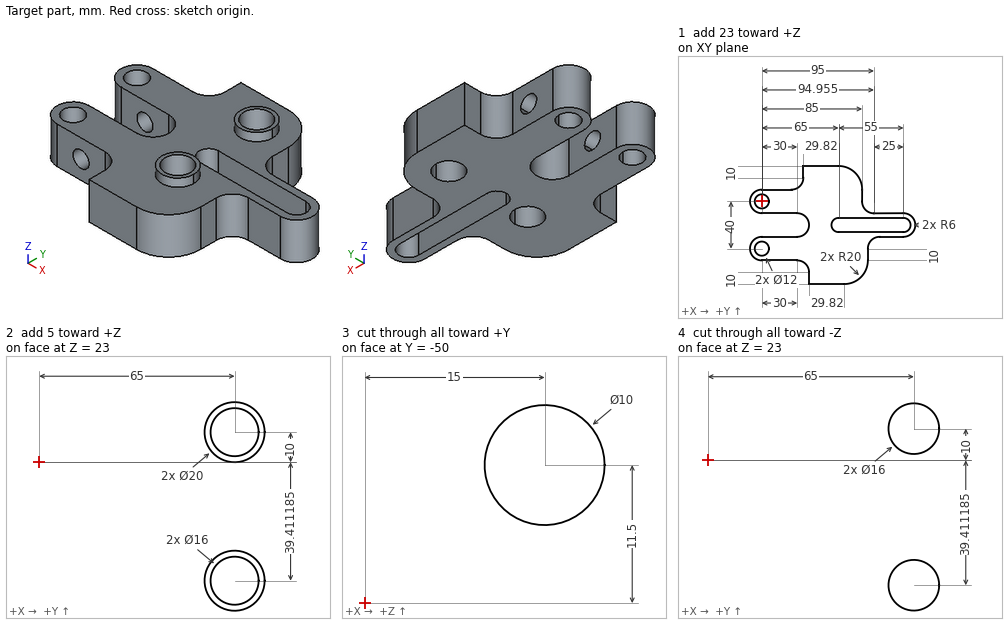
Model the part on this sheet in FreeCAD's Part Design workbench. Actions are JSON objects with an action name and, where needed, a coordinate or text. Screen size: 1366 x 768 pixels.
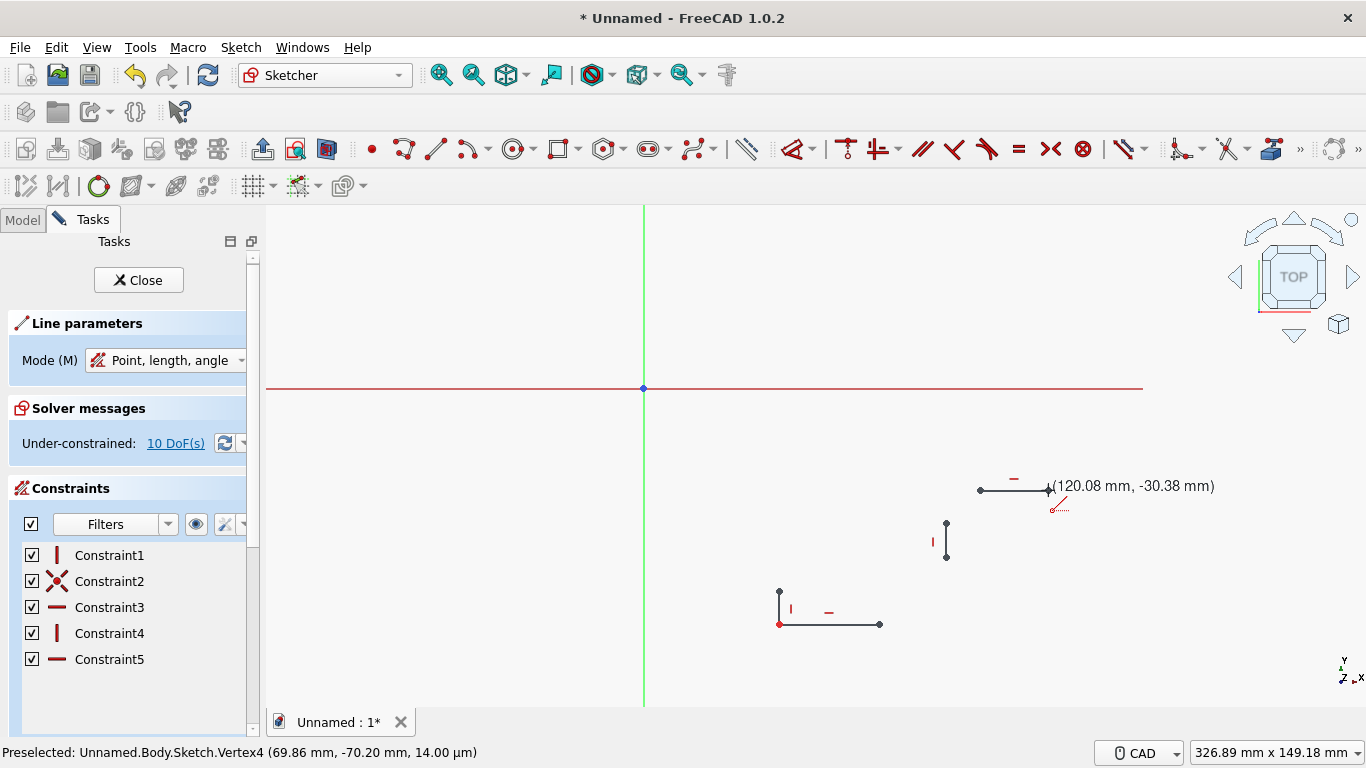
{"action": "left_click", "coordinate": [1048, 422]}
{"action": "left_click", "coordinate": [964, 427]}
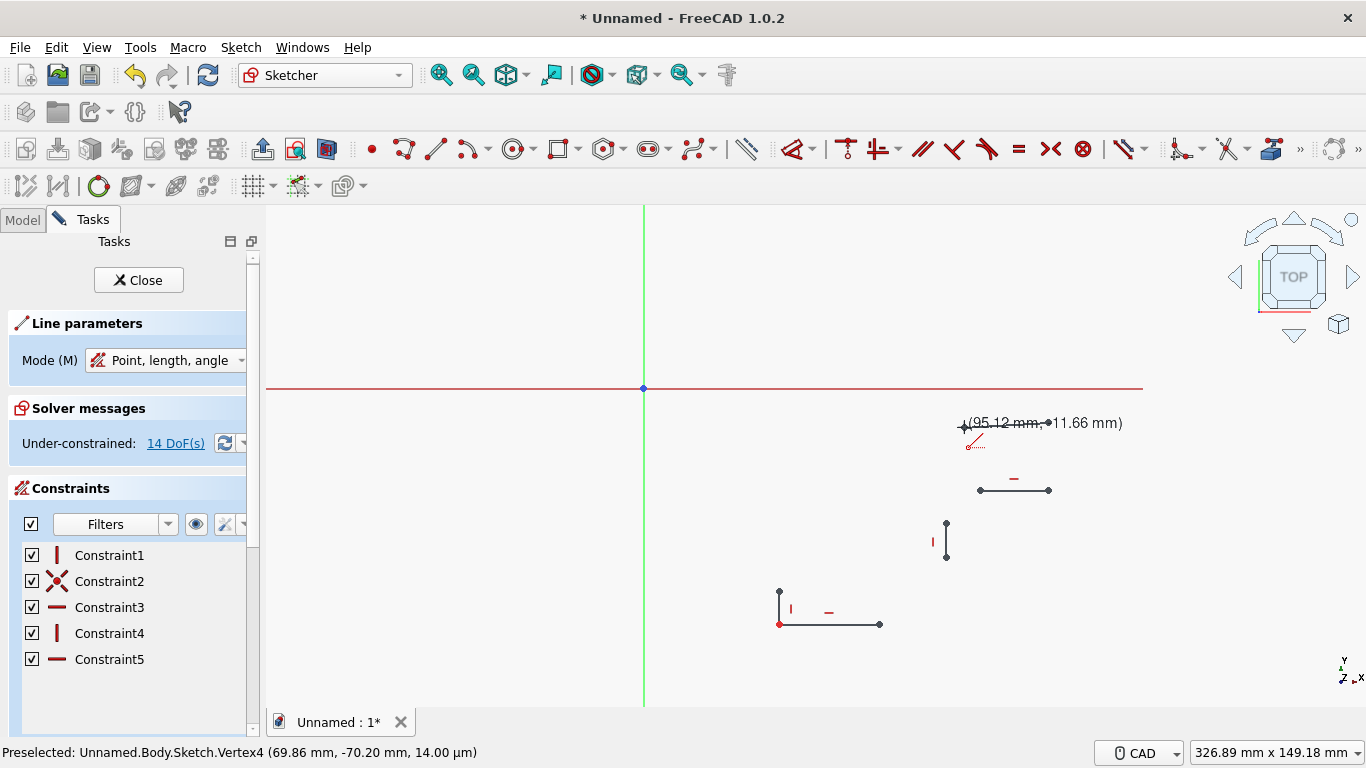
{"action": "scroll", "coordinate": [930, 389], "scroll_direction": "up", "scroll_amount": 22}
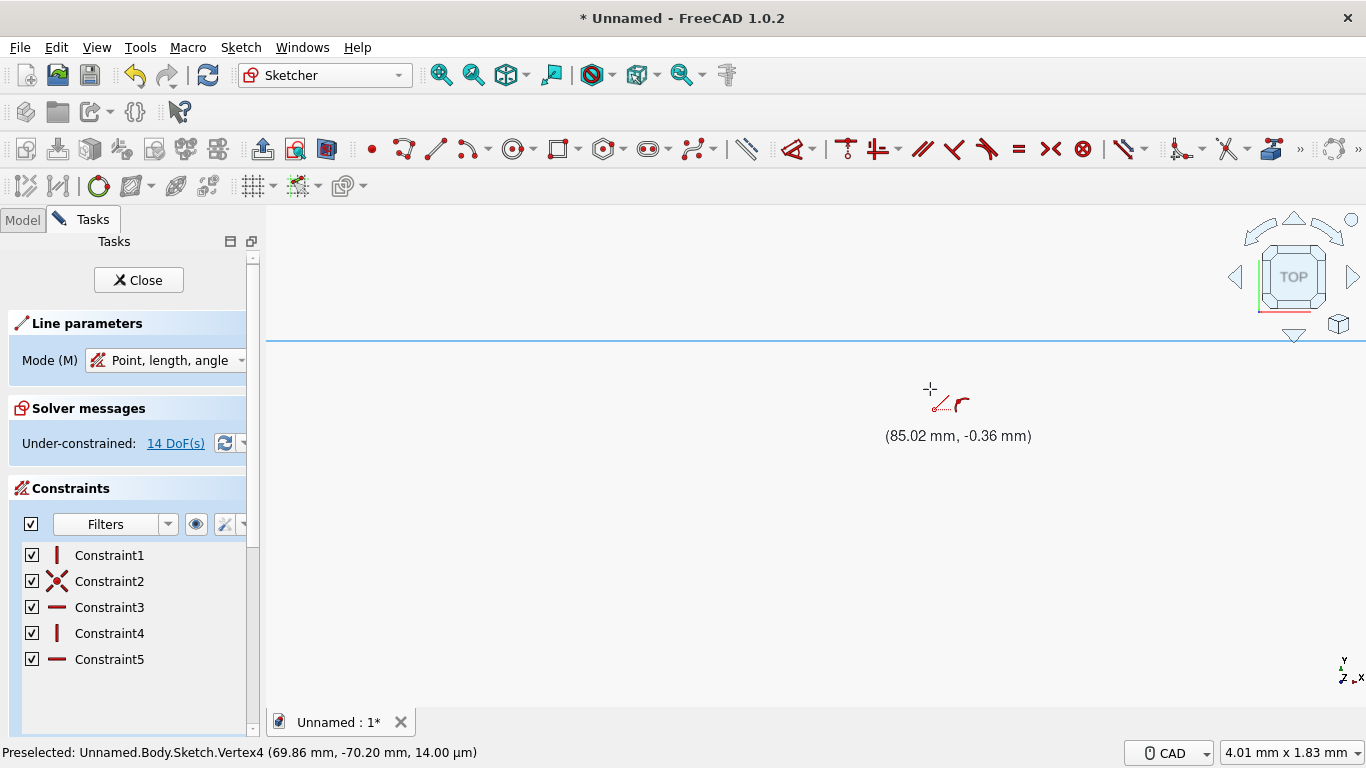
{"action": "left_click", "coordinate": [864, 360]}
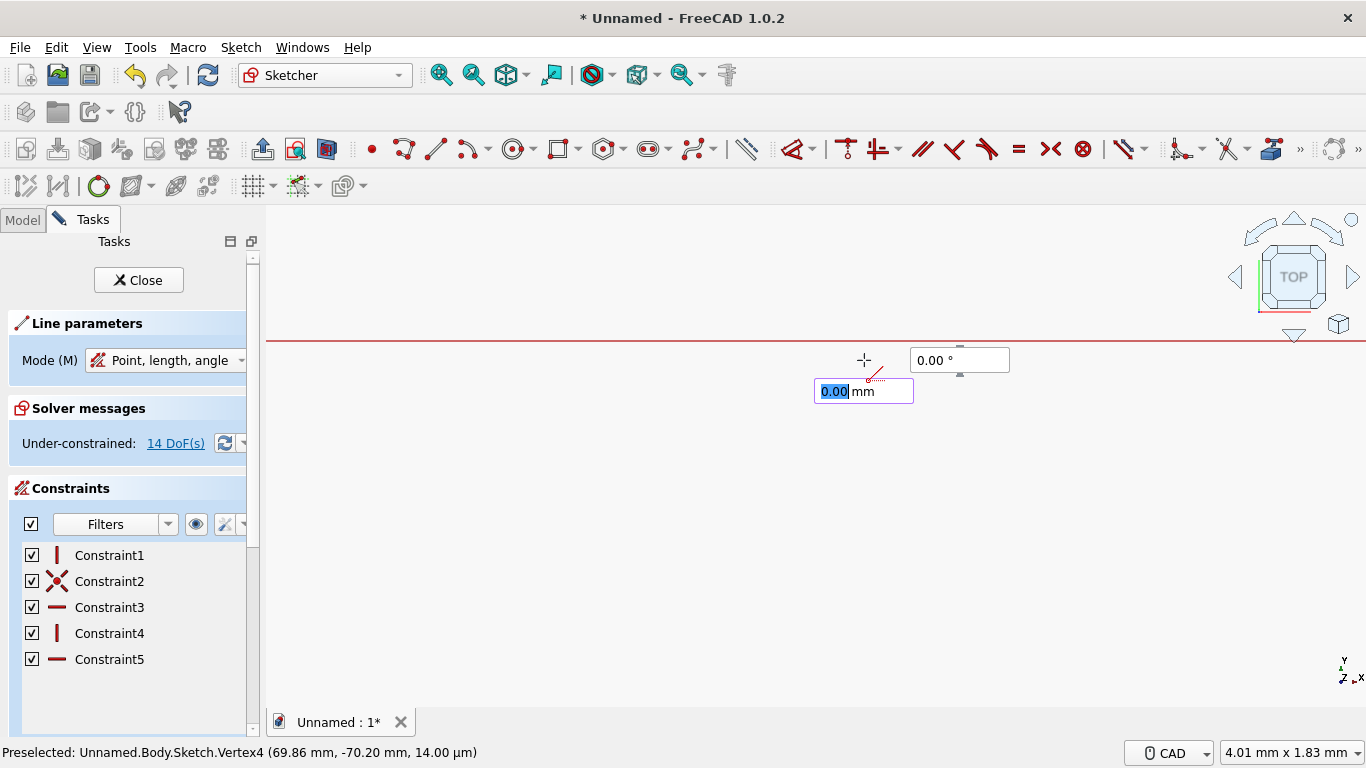
{"action": "scroll", "coordinate": [748, 456], "scroll_direction": "down", "scroll_amount": 15}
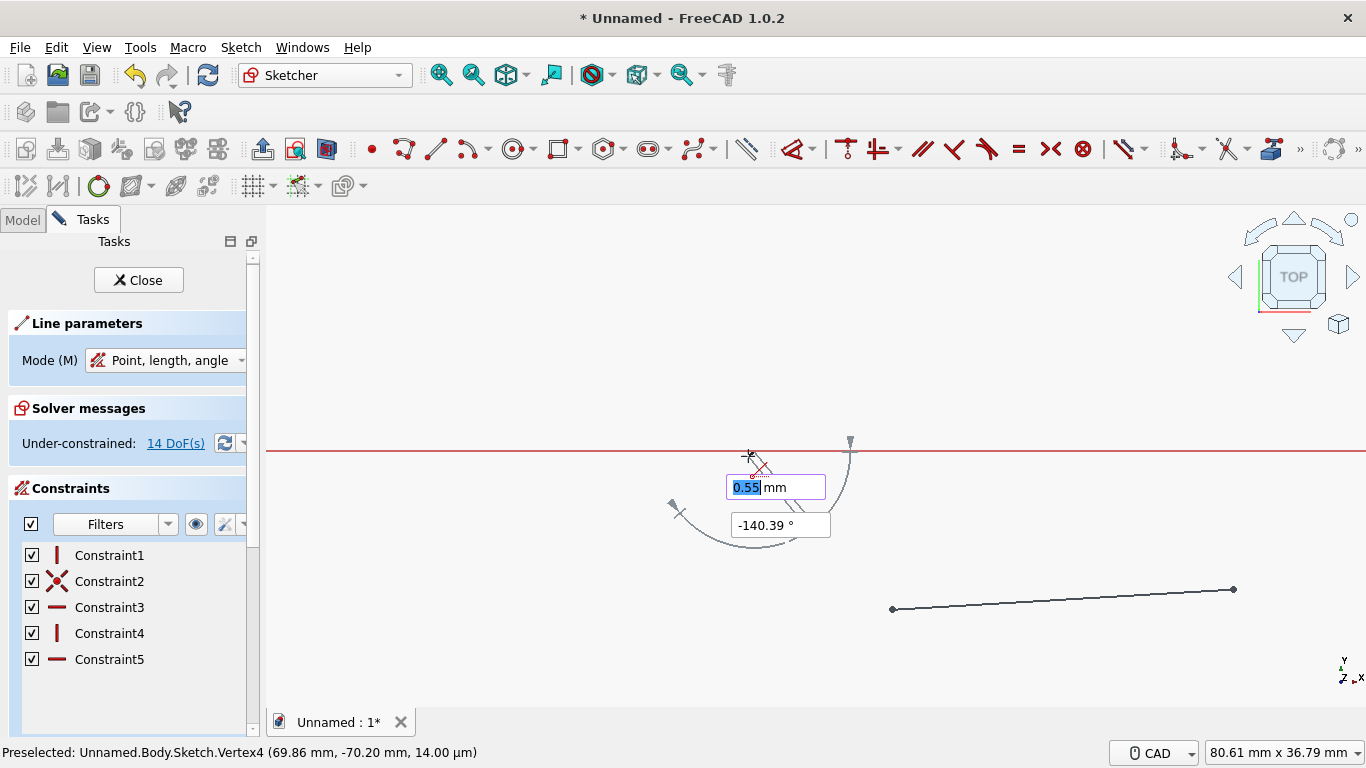
{"action": "scroll", "coordinate": [857, 368], "scroll_direction": "down", "scroll_amount": 7}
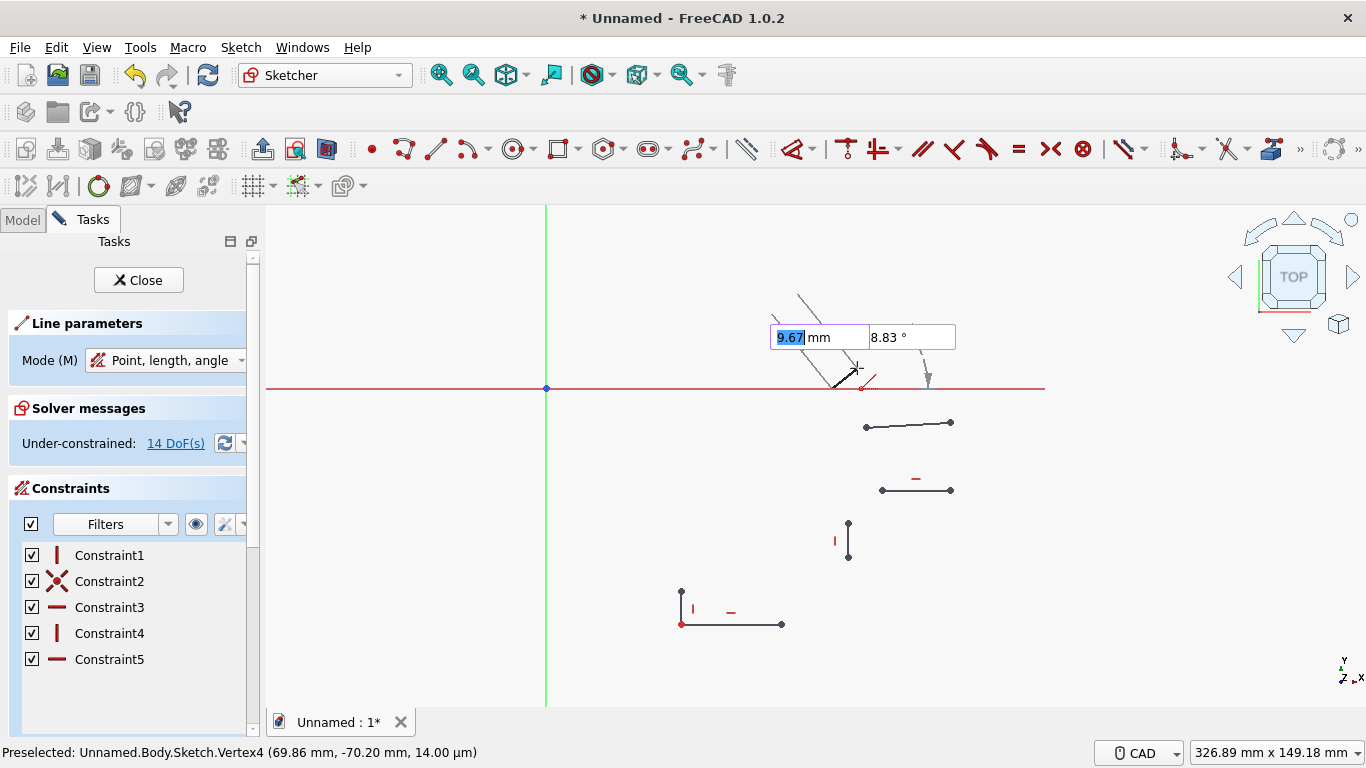
{"action": "left_click", "coordinate": [835, 355]}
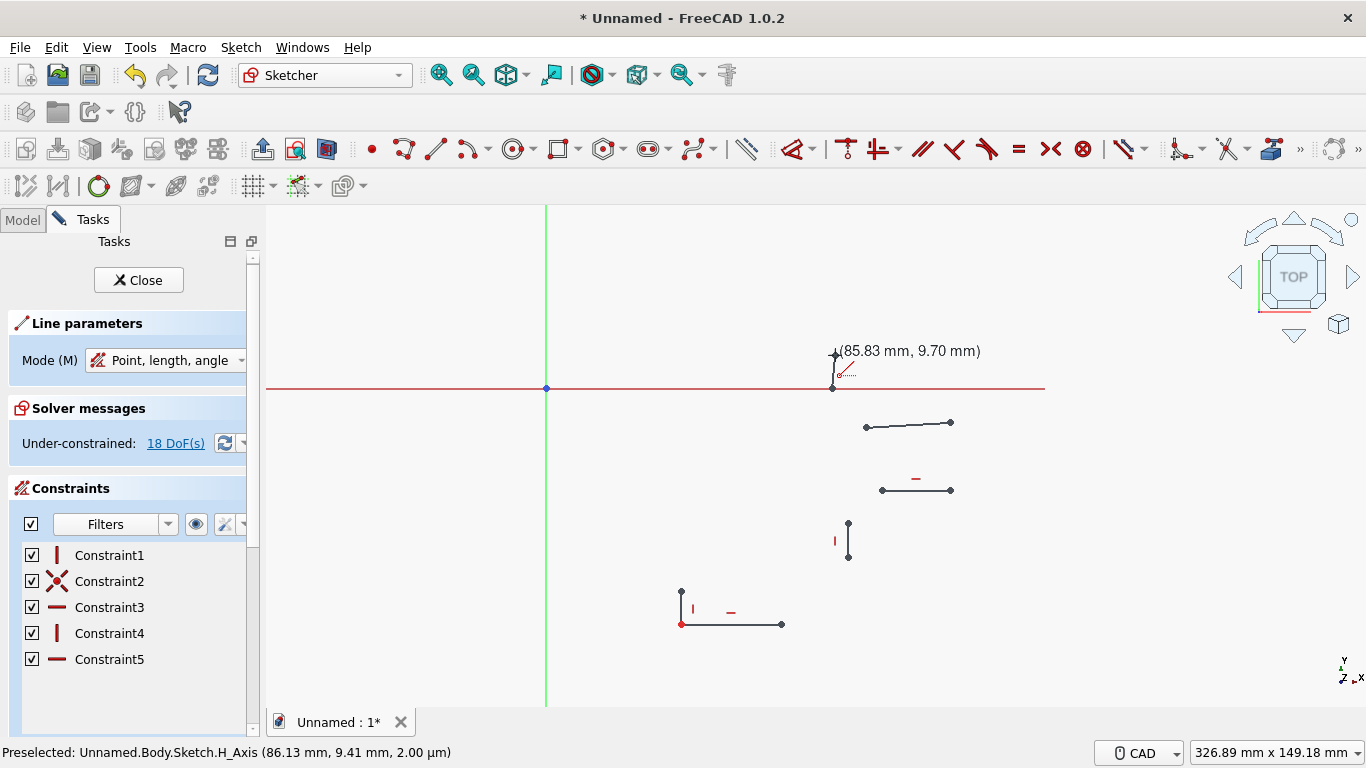
{"action": "left_click", "coordinate": [404, 150]}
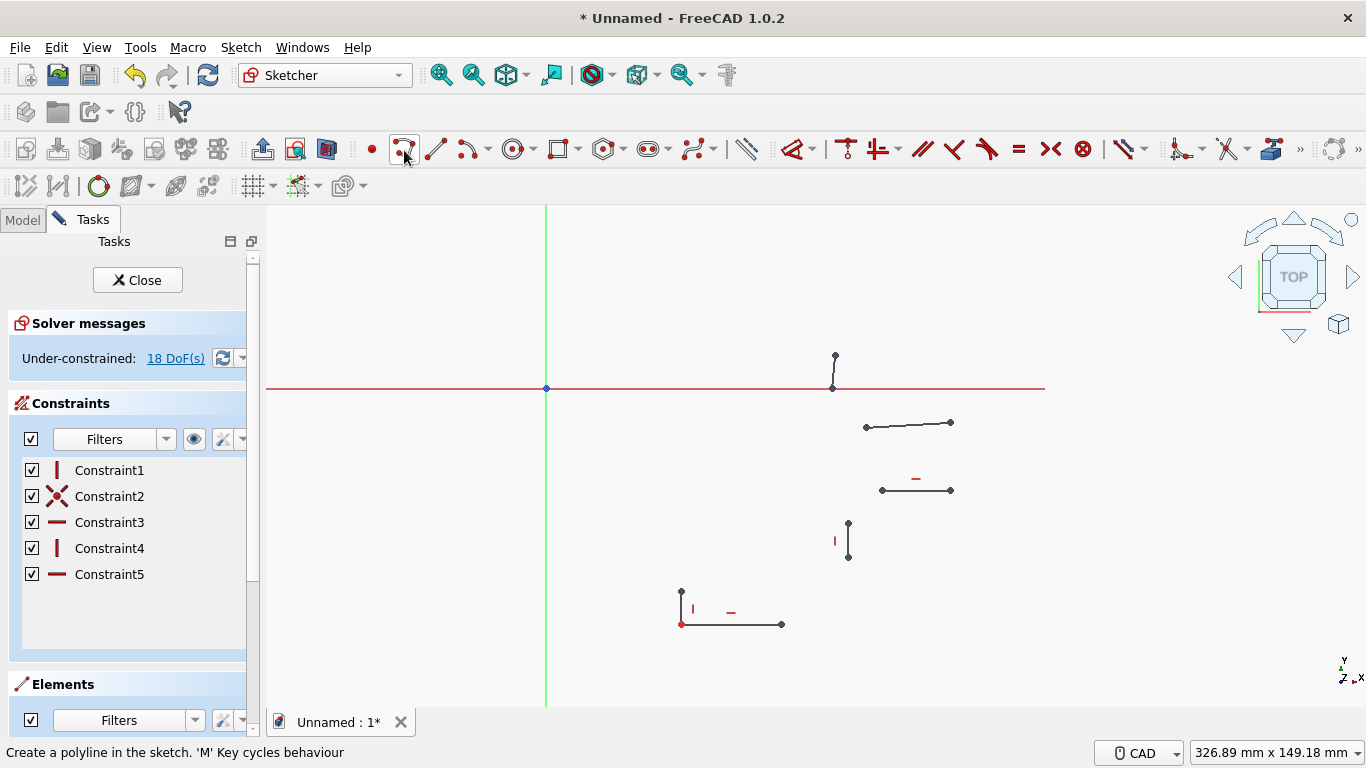
{"action": "left_click", "coordinate": [765, 288]}
{"action": "left_click", "coordinate": [665, 288]}
{"action": "left_click", "coordinate": [665, 321]}
{"action": "right_click", "coordinate": [665, 321]}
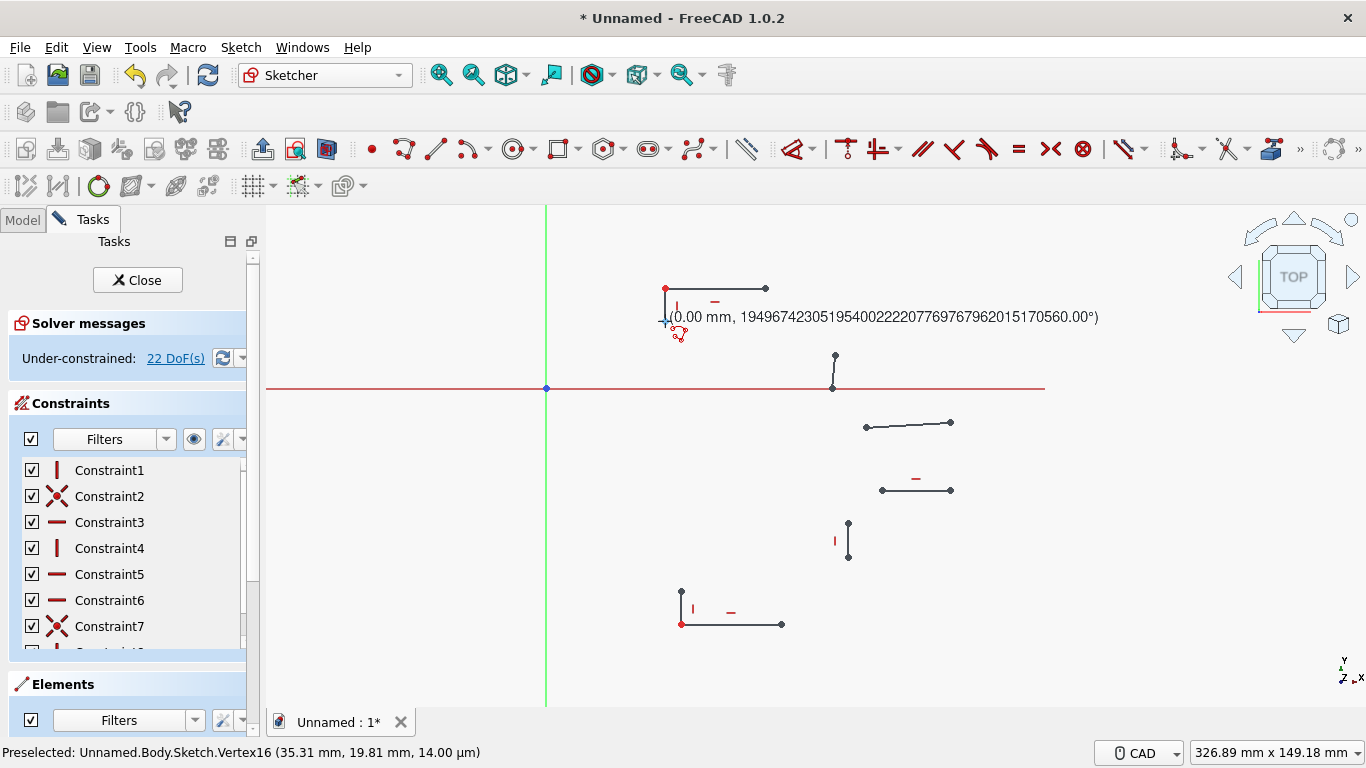
{"action": "left_click", "coordinate": [436, 150]}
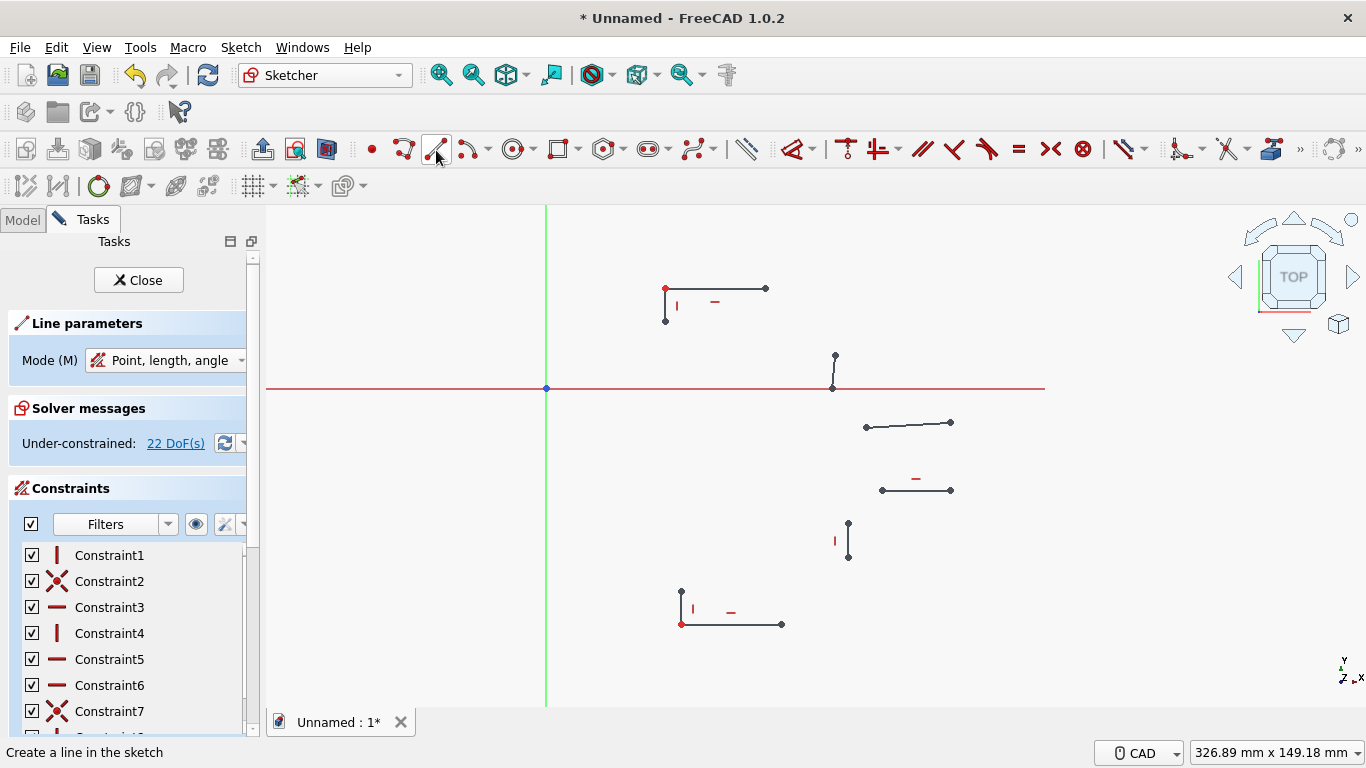
{"action": "left_click", "coordinate": [631, 355]}
{"action": "left_click", "coordinate": [546, 355]}